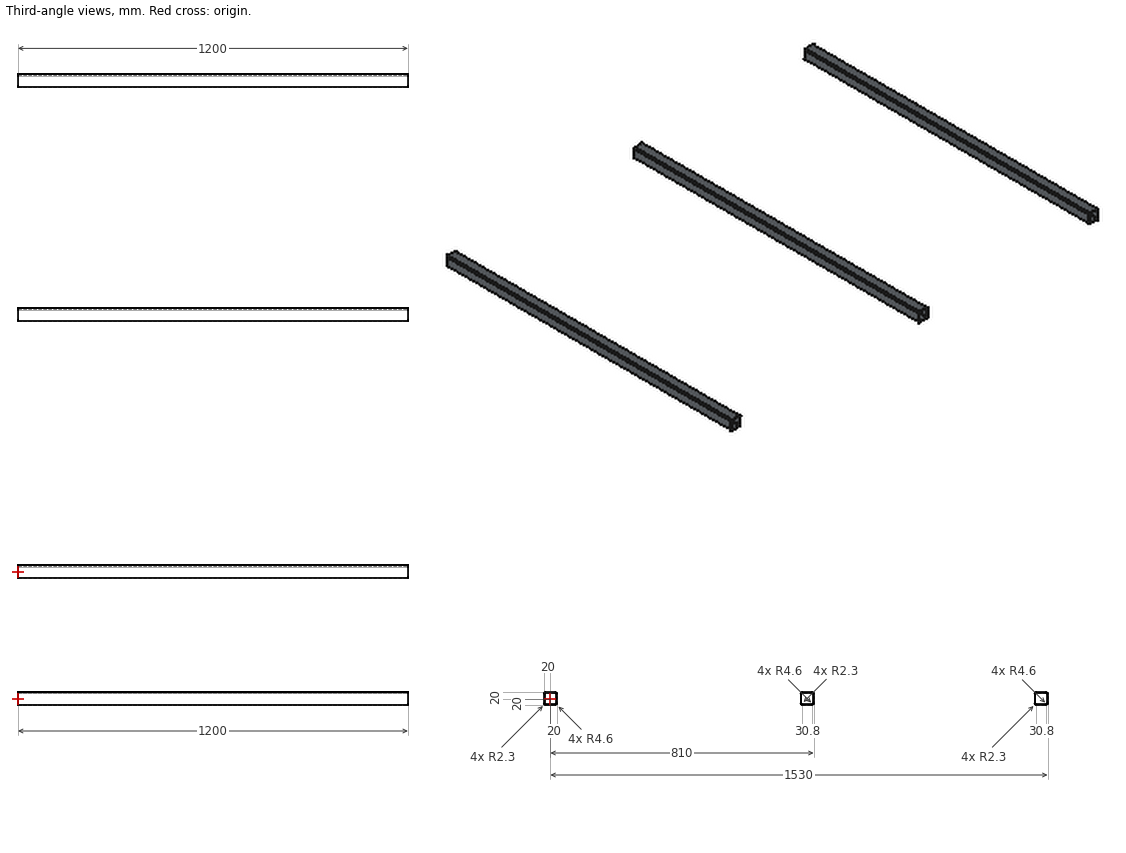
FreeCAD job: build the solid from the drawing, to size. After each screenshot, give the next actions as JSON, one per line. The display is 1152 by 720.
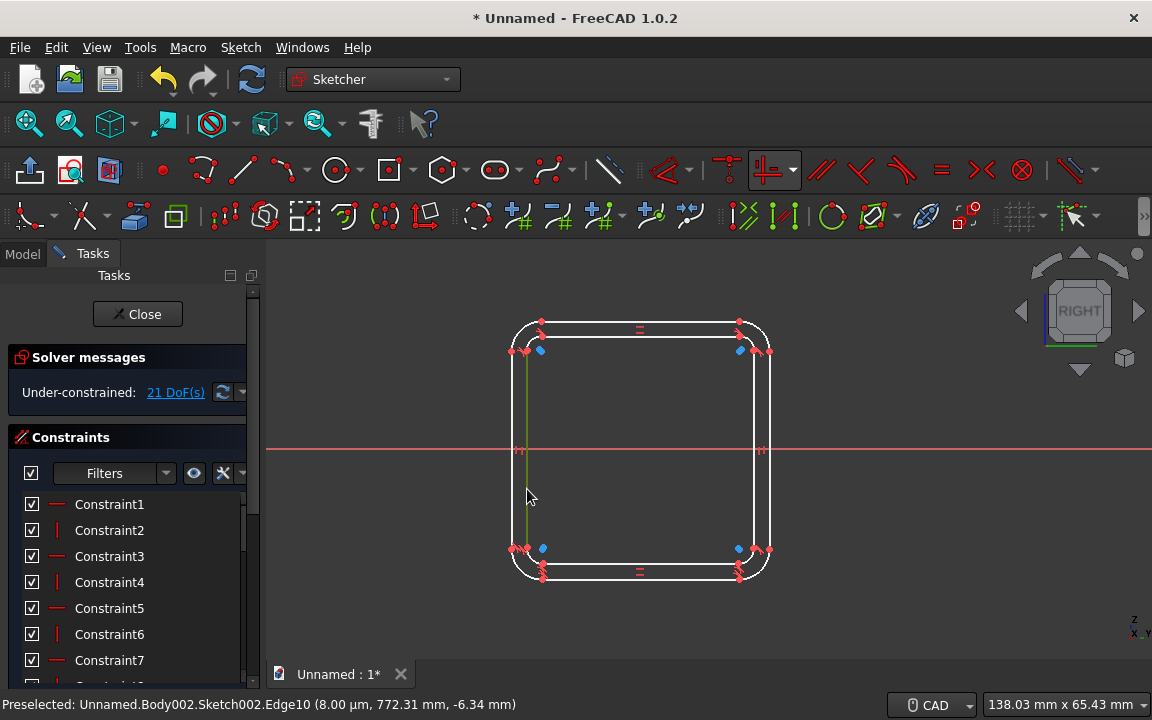
{"action": "left_click", "coordinate": [531, 340]}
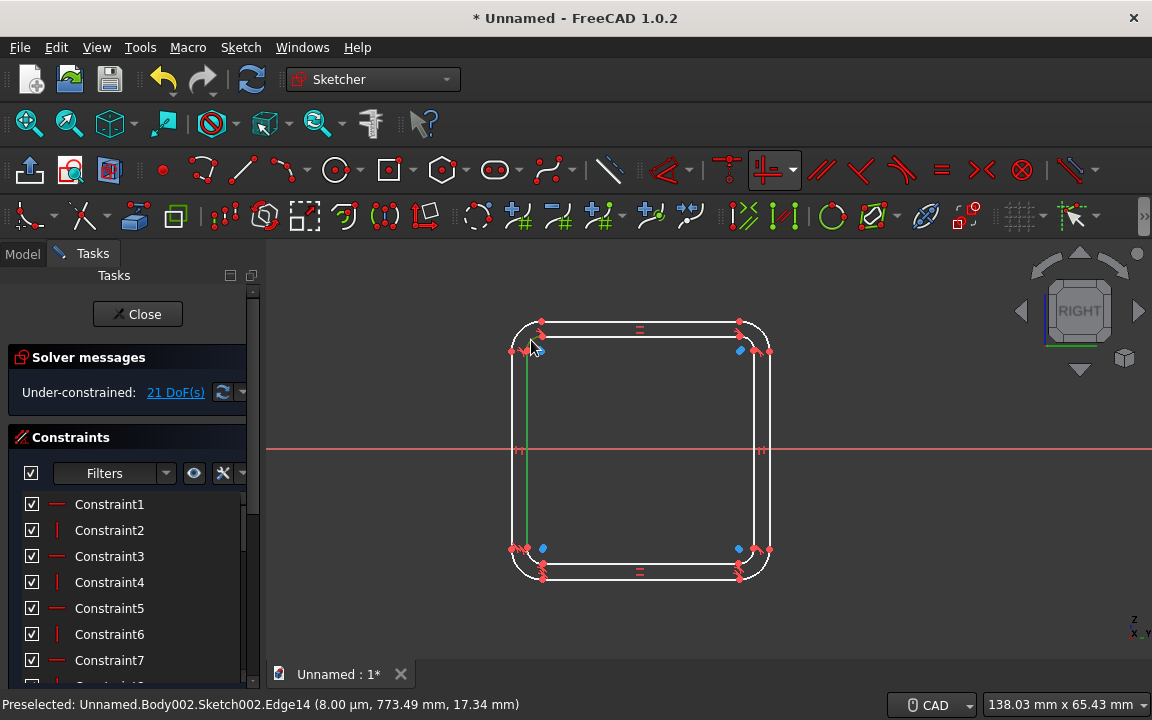
{"action": "key", "text": "t"}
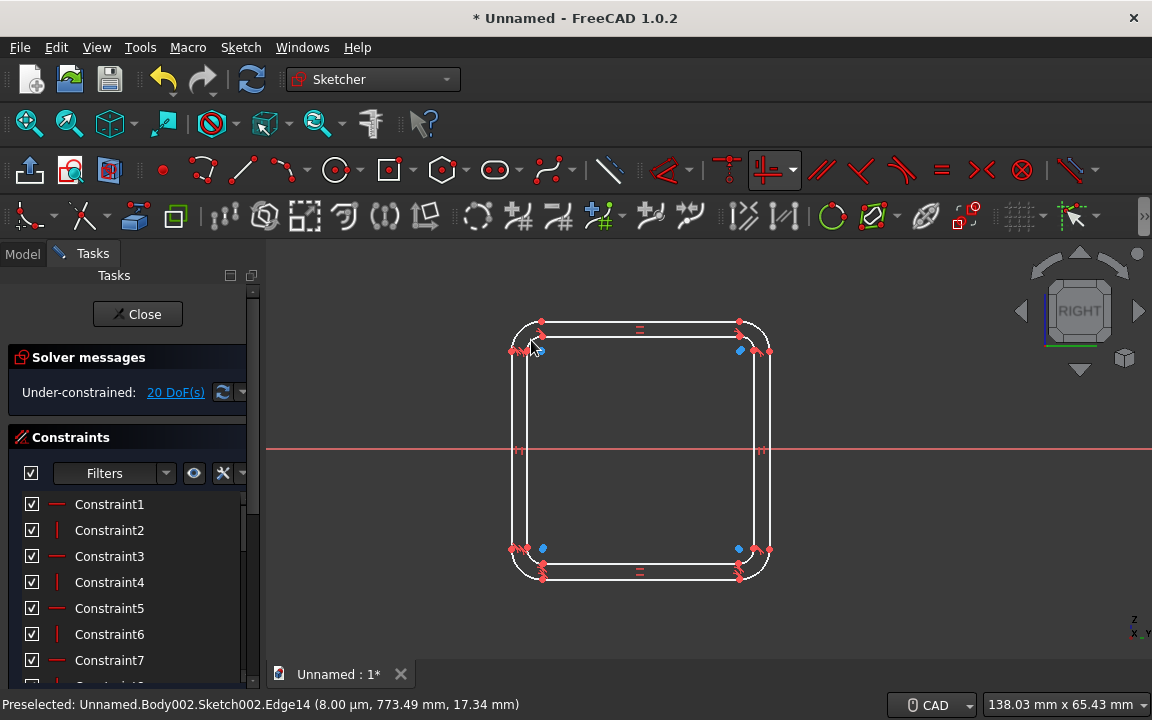
{"action": "left_click", "coordinate": [601, 337]}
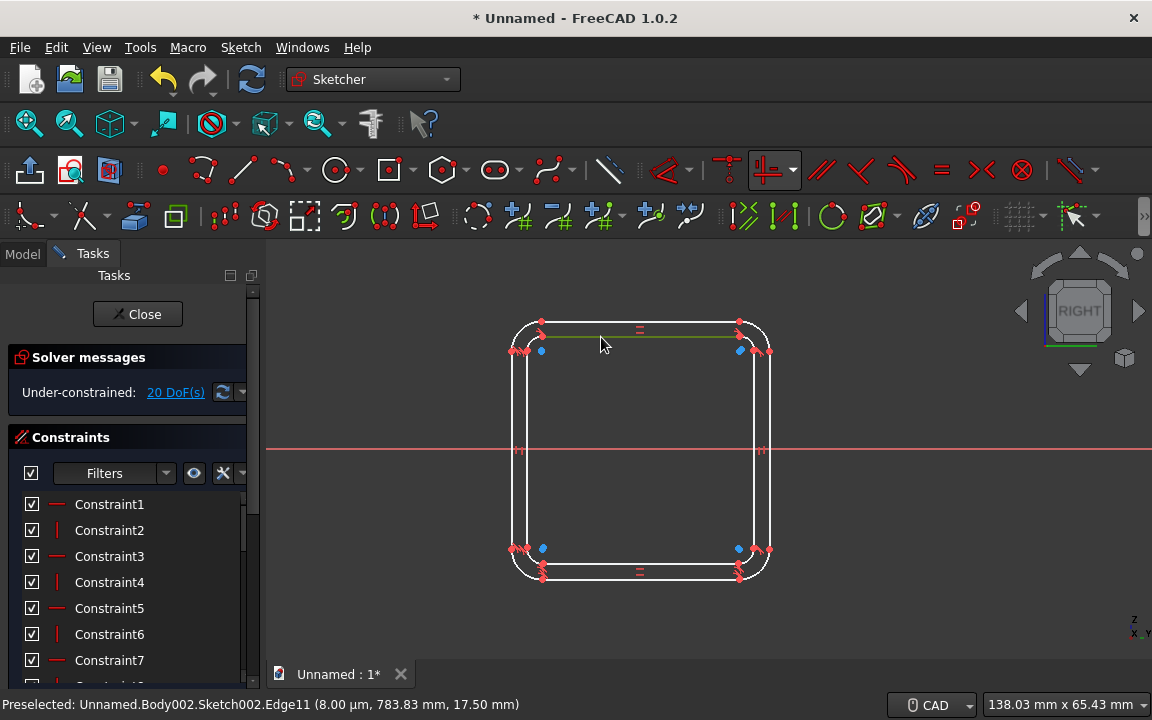
{"action": "scroll", "coordinate": [531, 341], "scroll_direction": "up", "scroll_amount": 2}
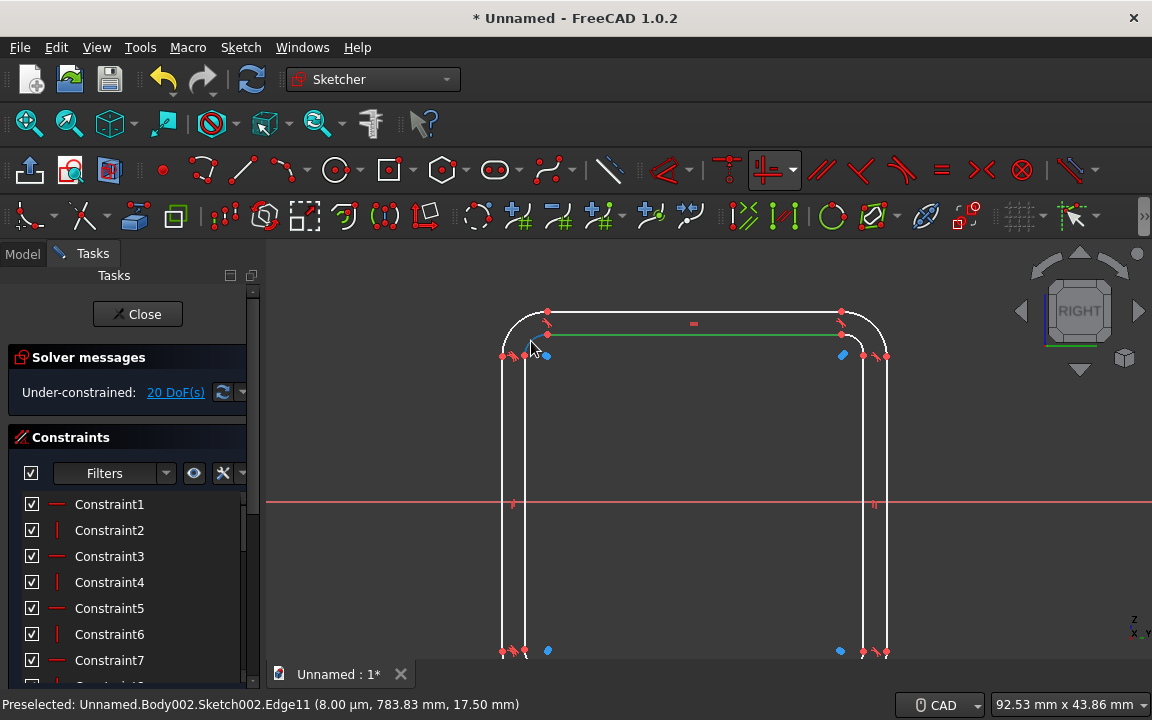
{"action": "left_click", "coordinate": [532, 340]}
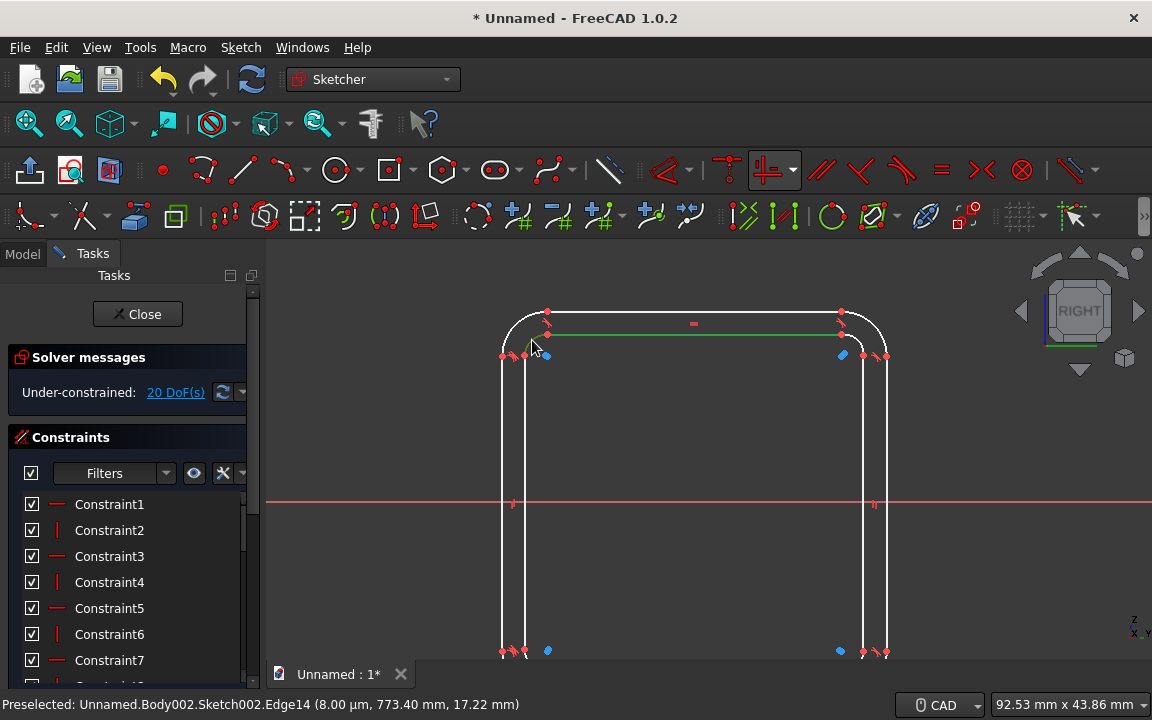
{"action": "key", "text": "t"}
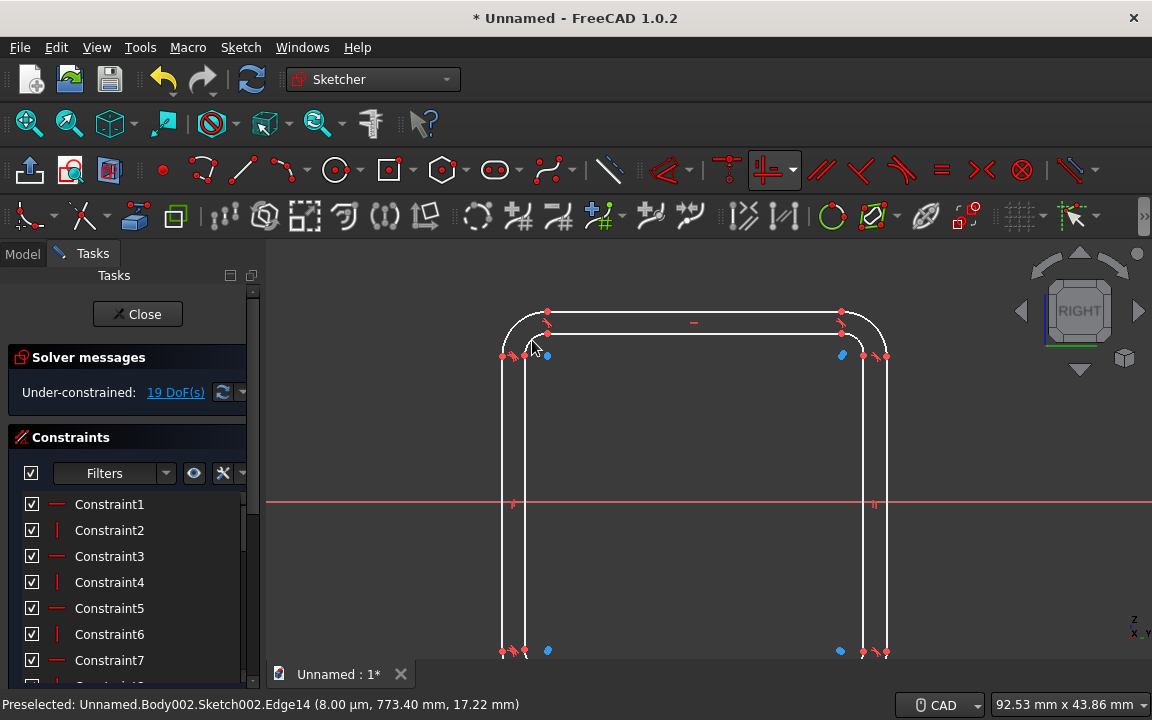
{"action": "left_click", "coordinate": [635, 333]}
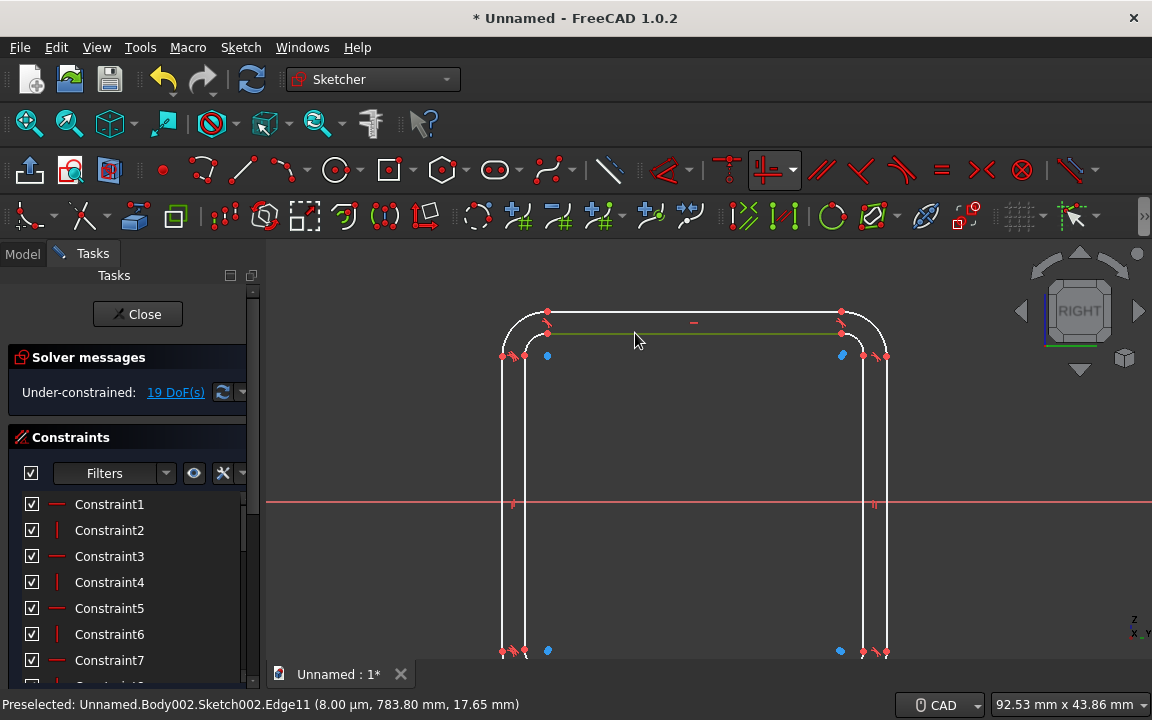
{"action": "scroll", "coordinate": [862, 345], "scroll_direction": "up", "scroll_amount": 2}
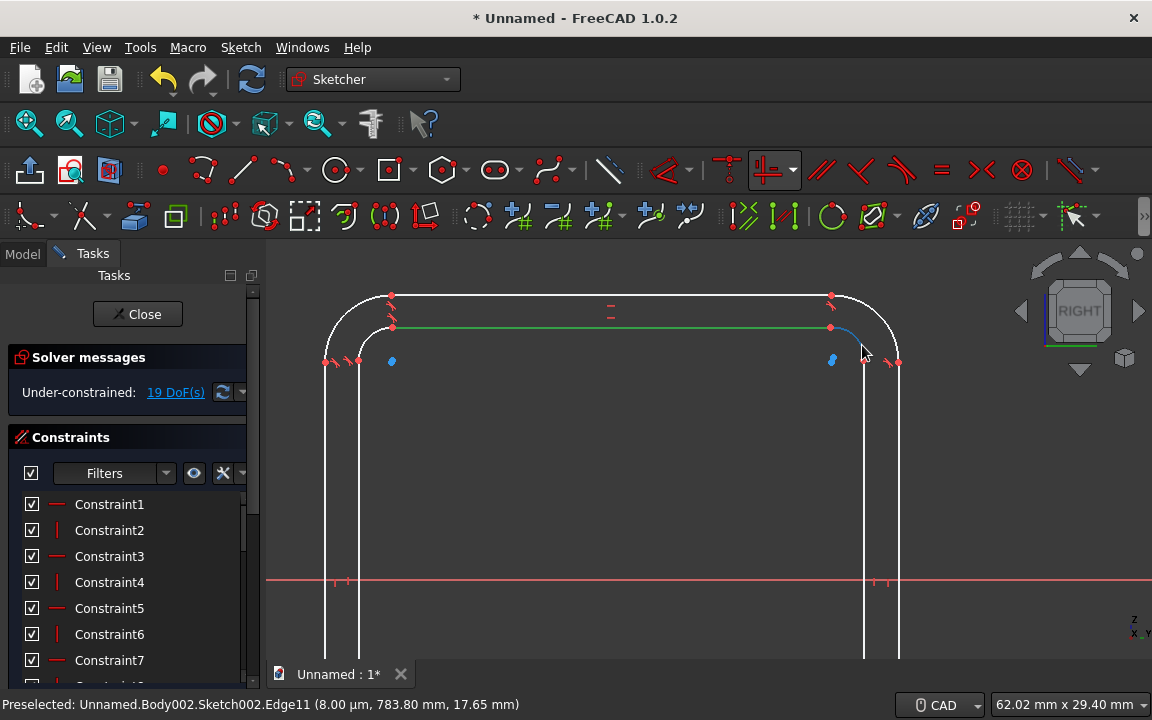
{"action": "left_click", "coordinate": [861, 345]}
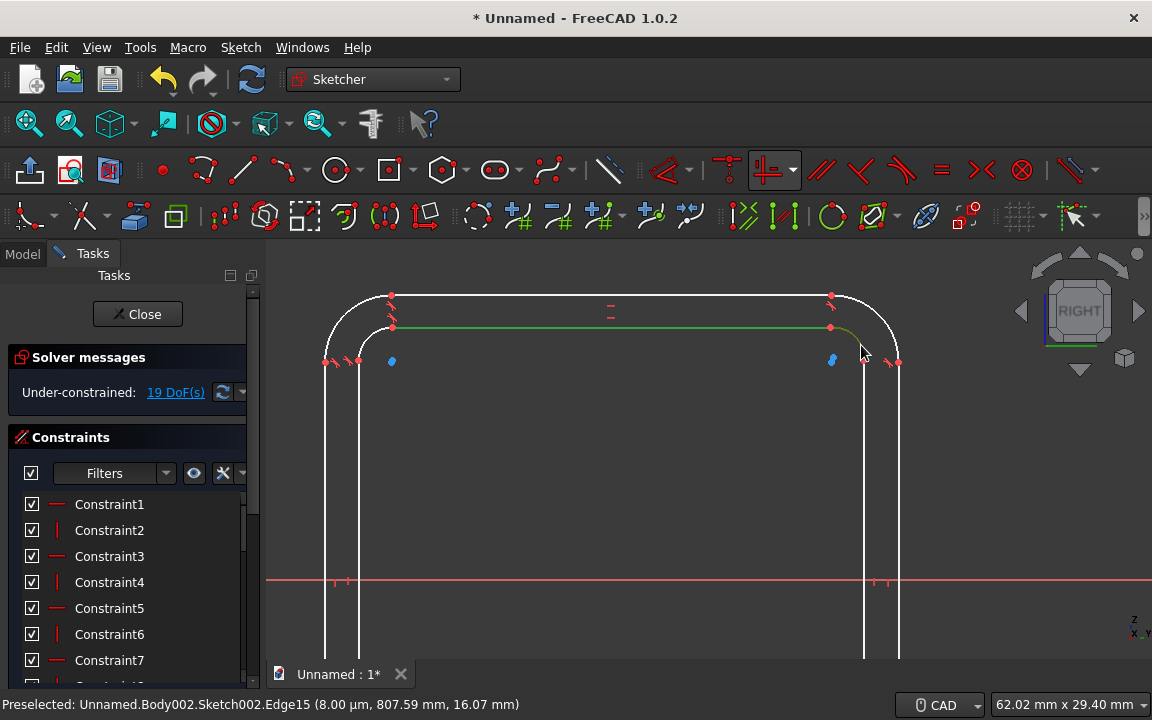
{"action": "left_click", "coordinate": [902, 170]}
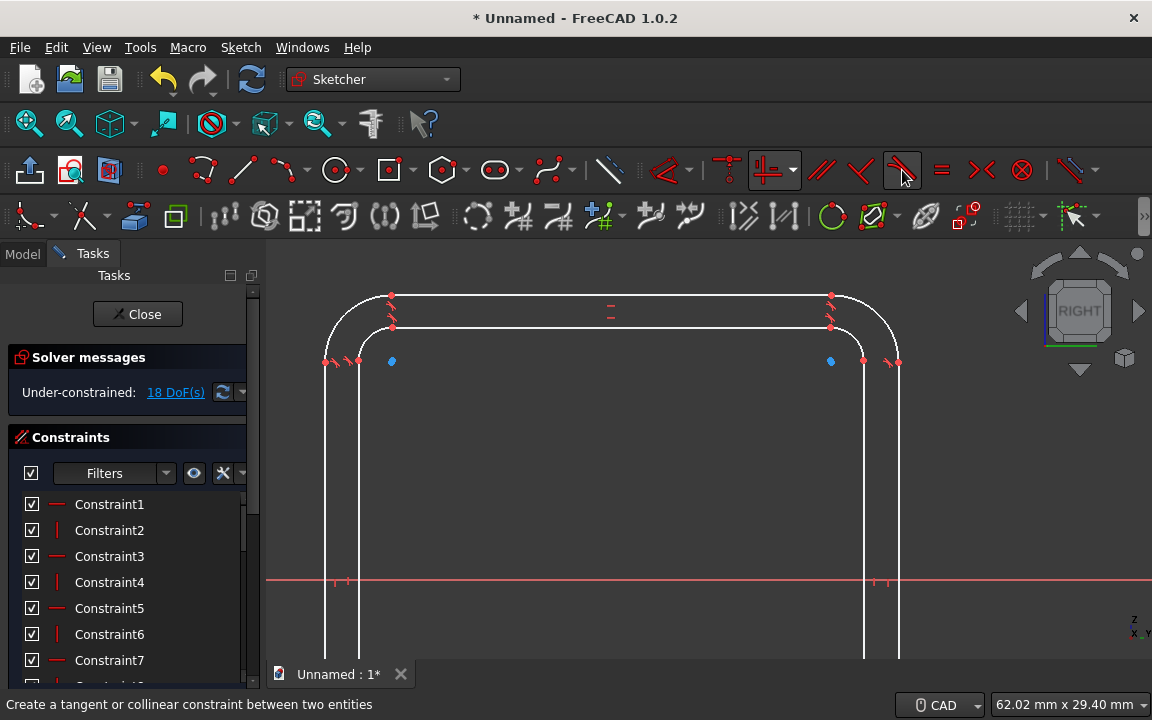
{"action": "left_click", "coordinate": [864, 493]}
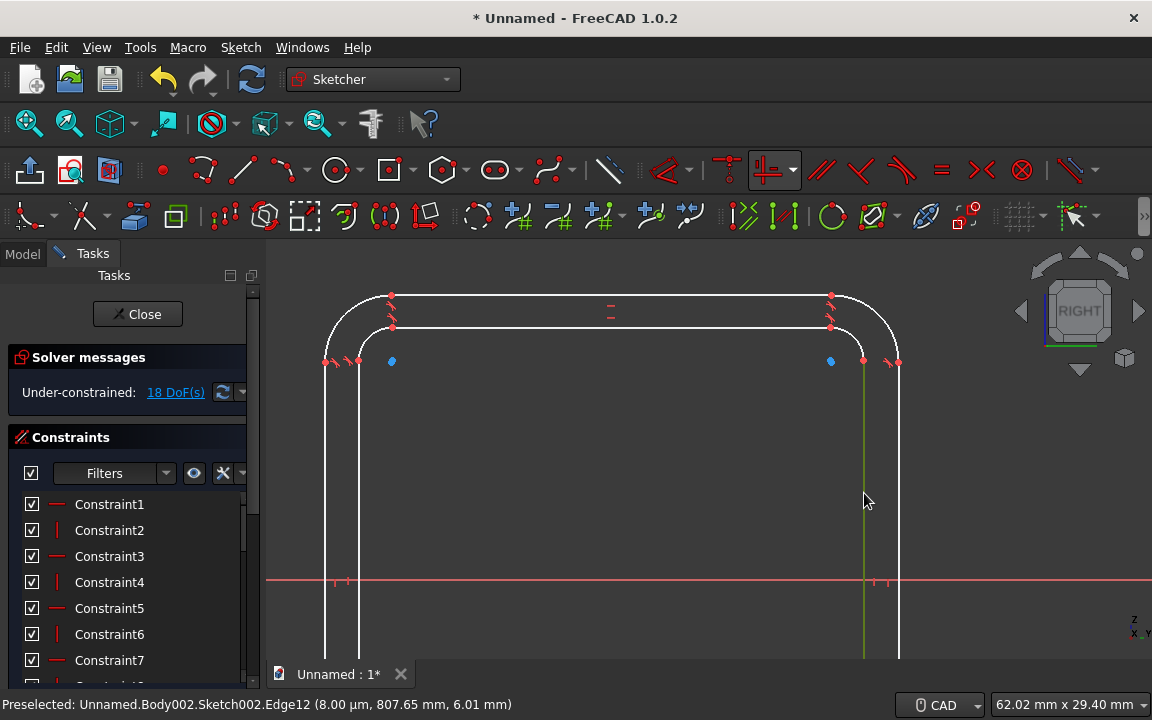
{"action": "left_click", "coordinate": [860, 346]}